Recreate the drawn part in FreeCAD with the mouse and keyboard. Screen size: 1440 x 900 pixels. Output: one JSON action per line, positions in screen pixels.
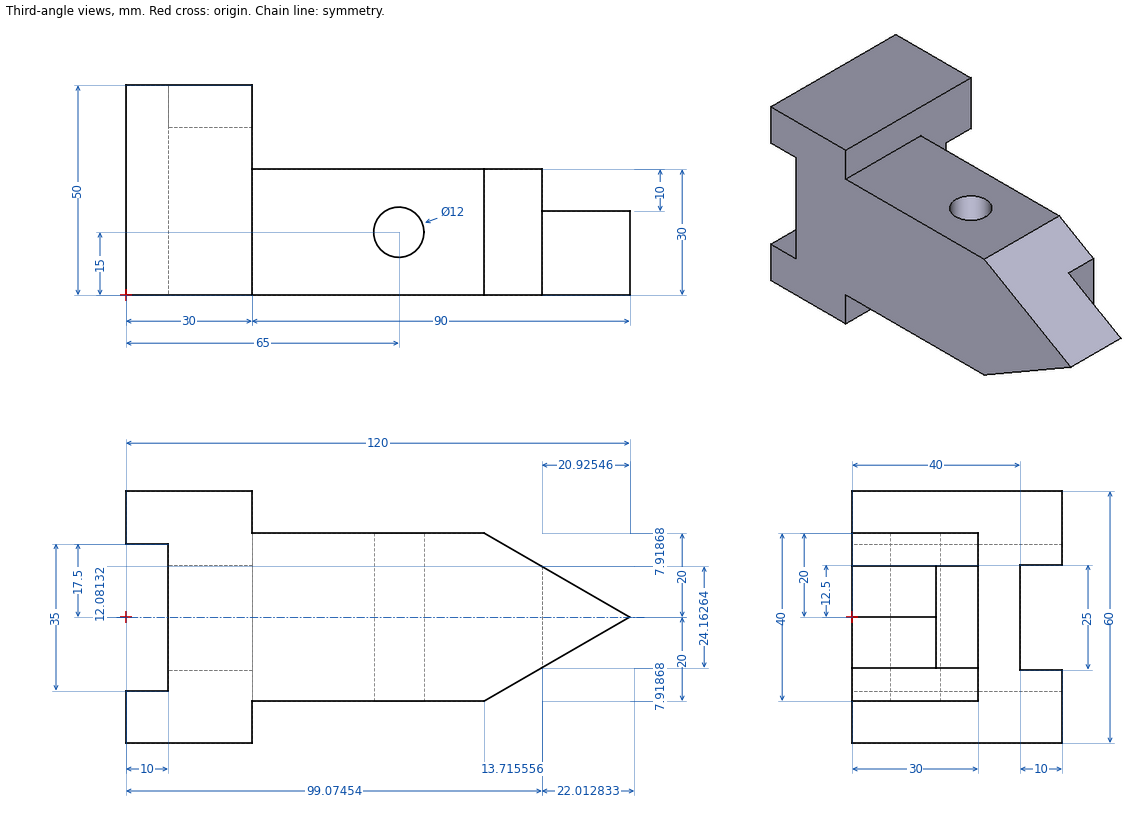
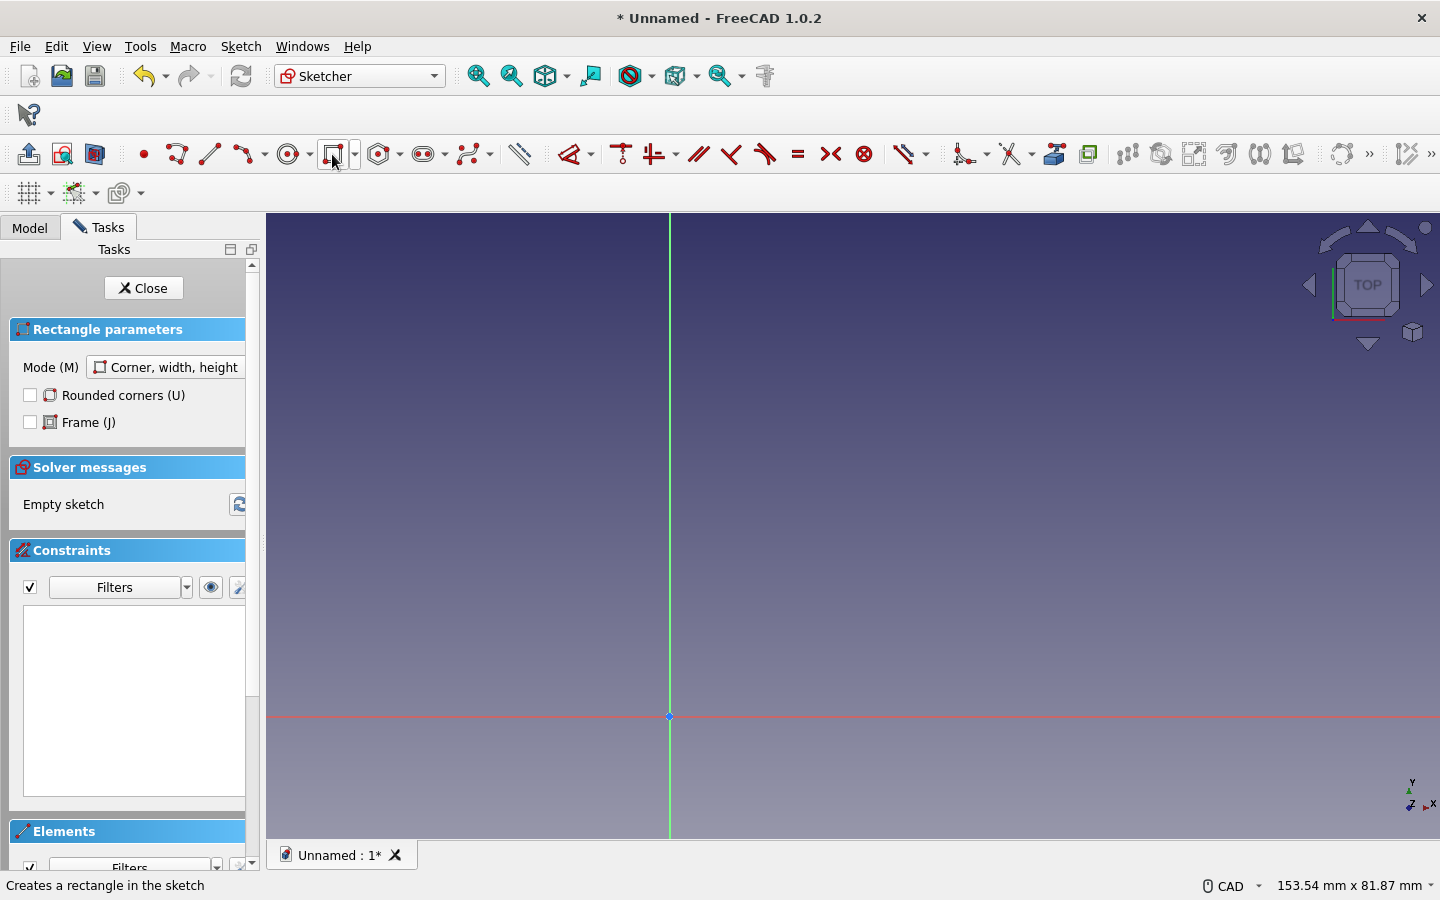
{"action": "left_click", "coordinate": [670, 717]}
{"action": "left_click", "coordinate": [899, 335]}
{"action": "key", "text": "Escape"}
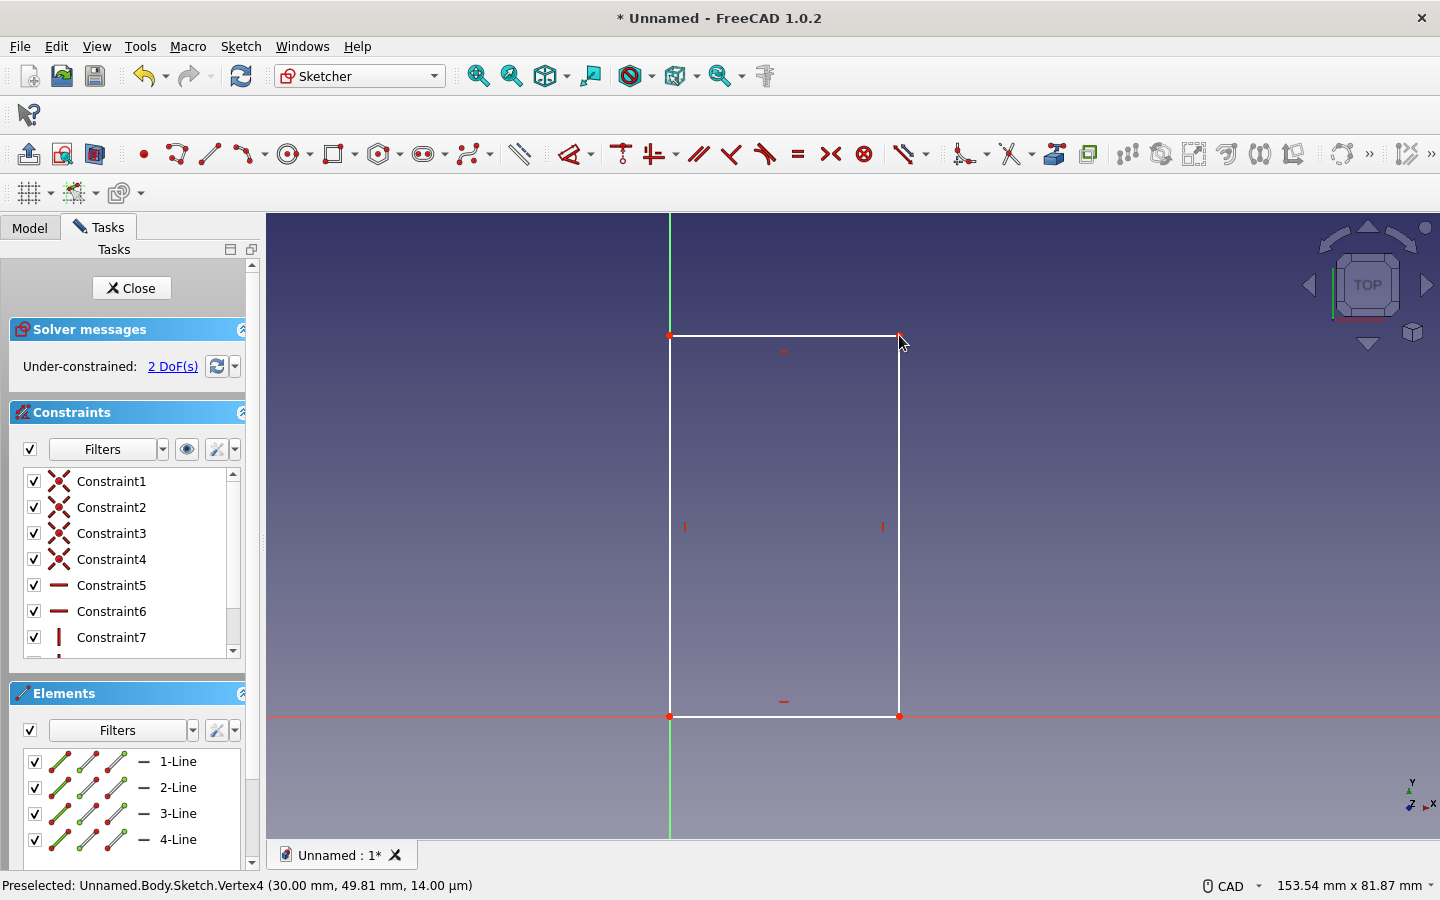
{"action": "left_click", "coordinate": [738, 717]}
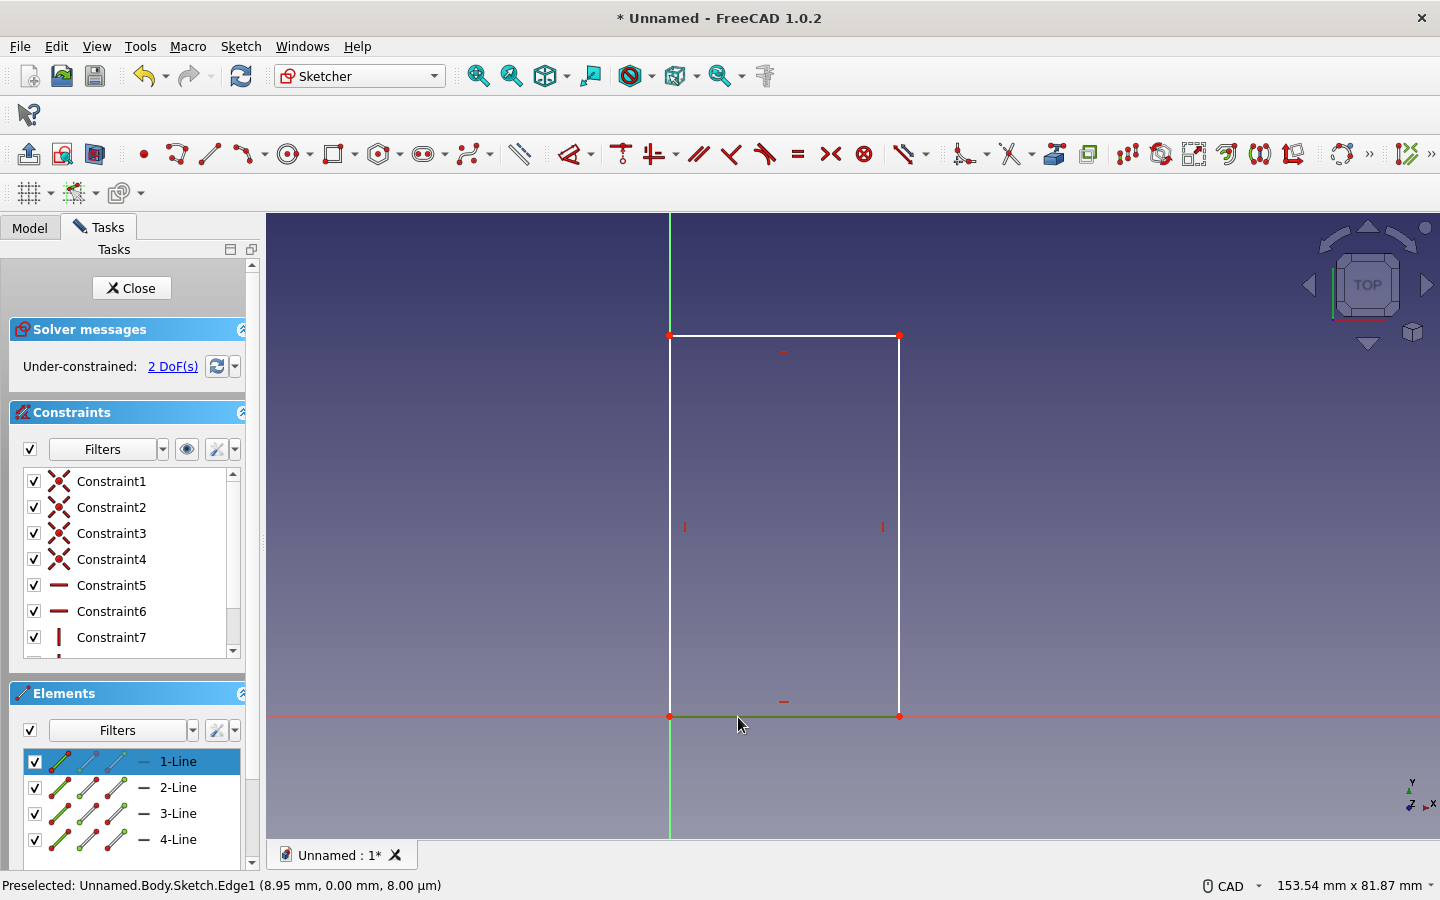
{"action": "left_click", "coordinate": [590, 154]}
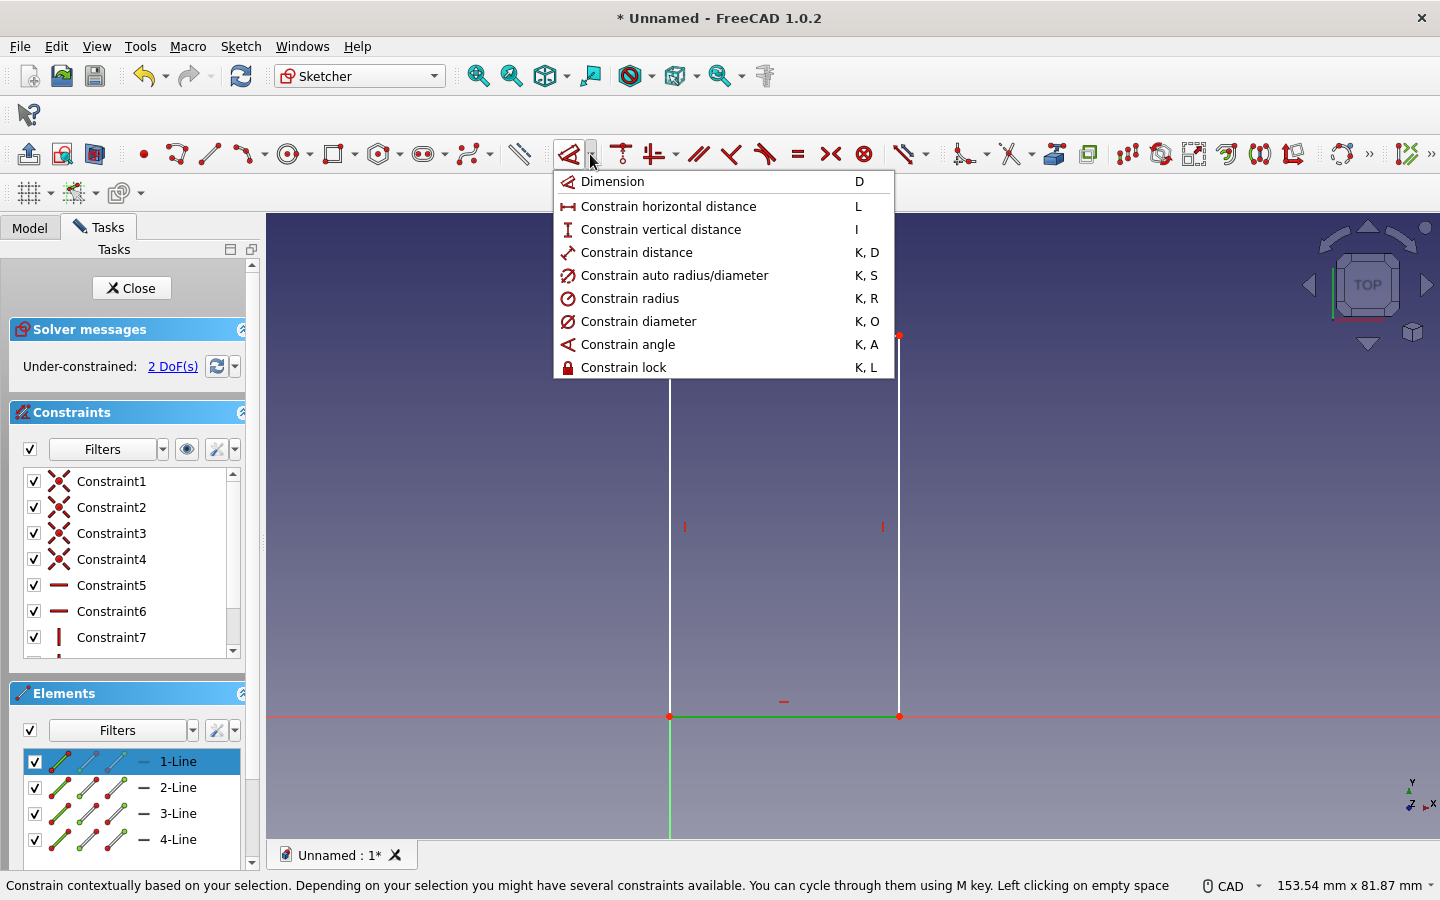
{"action": "left_click", "coordinate": [724, 206]}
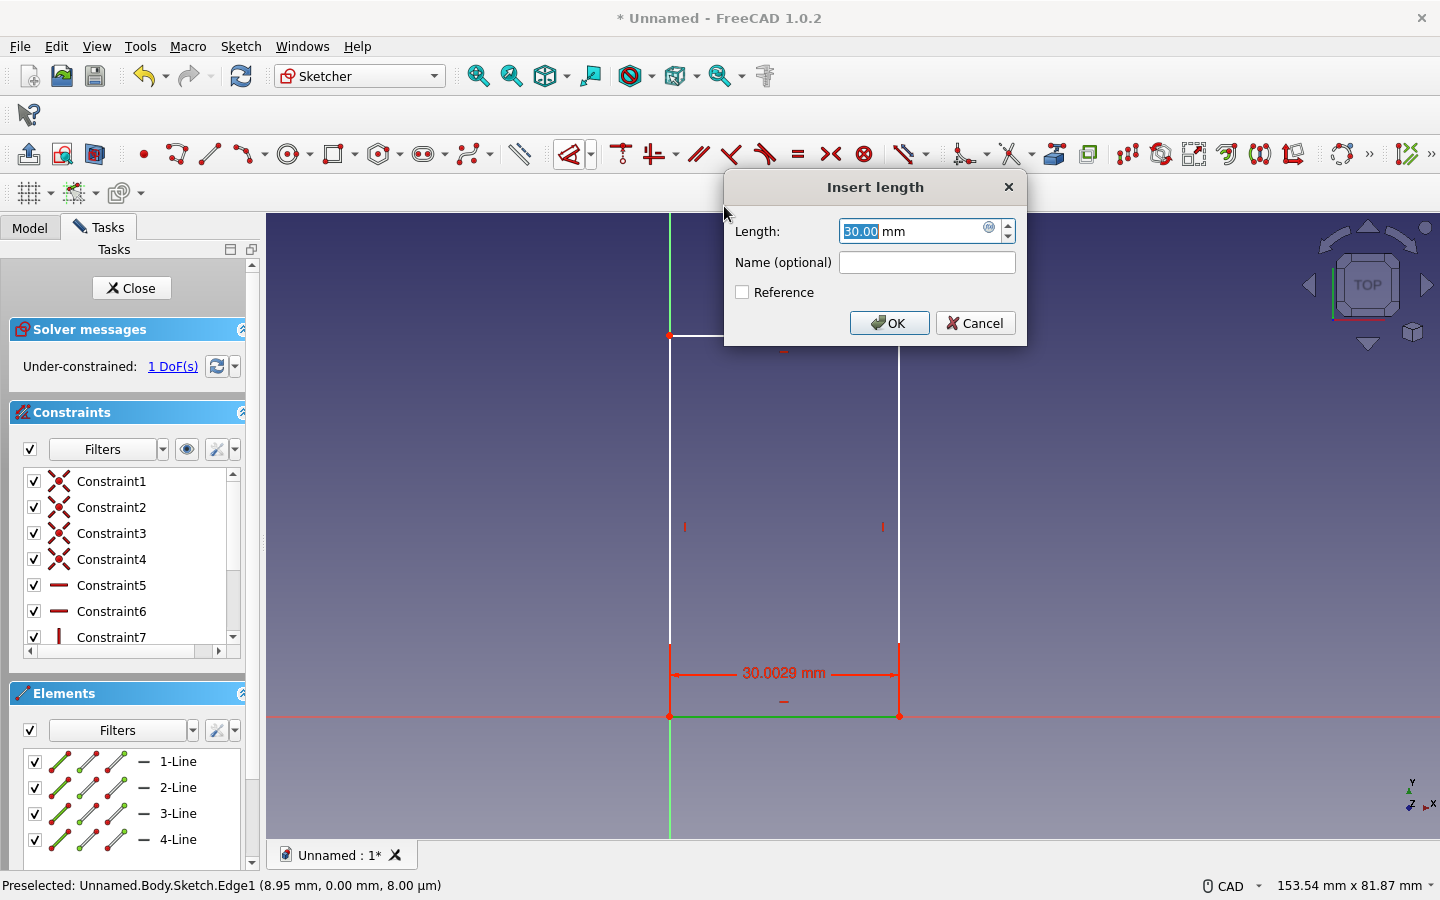
{"action": "type", "text": "30"}
{"action": "key", "text": "Return"}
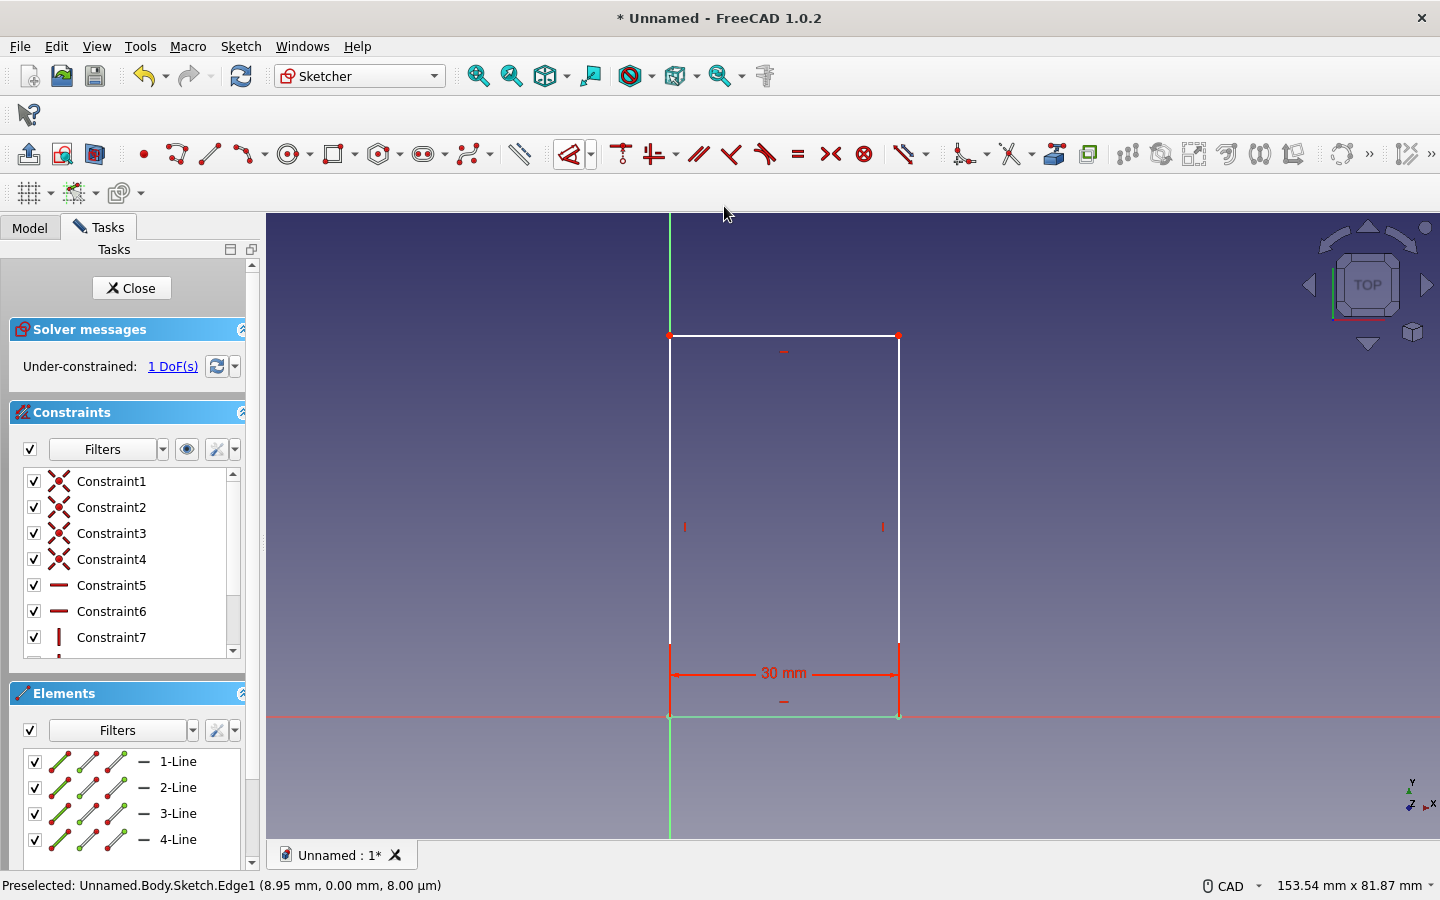
{"action": "left_click", "coordinate": [899, 603]}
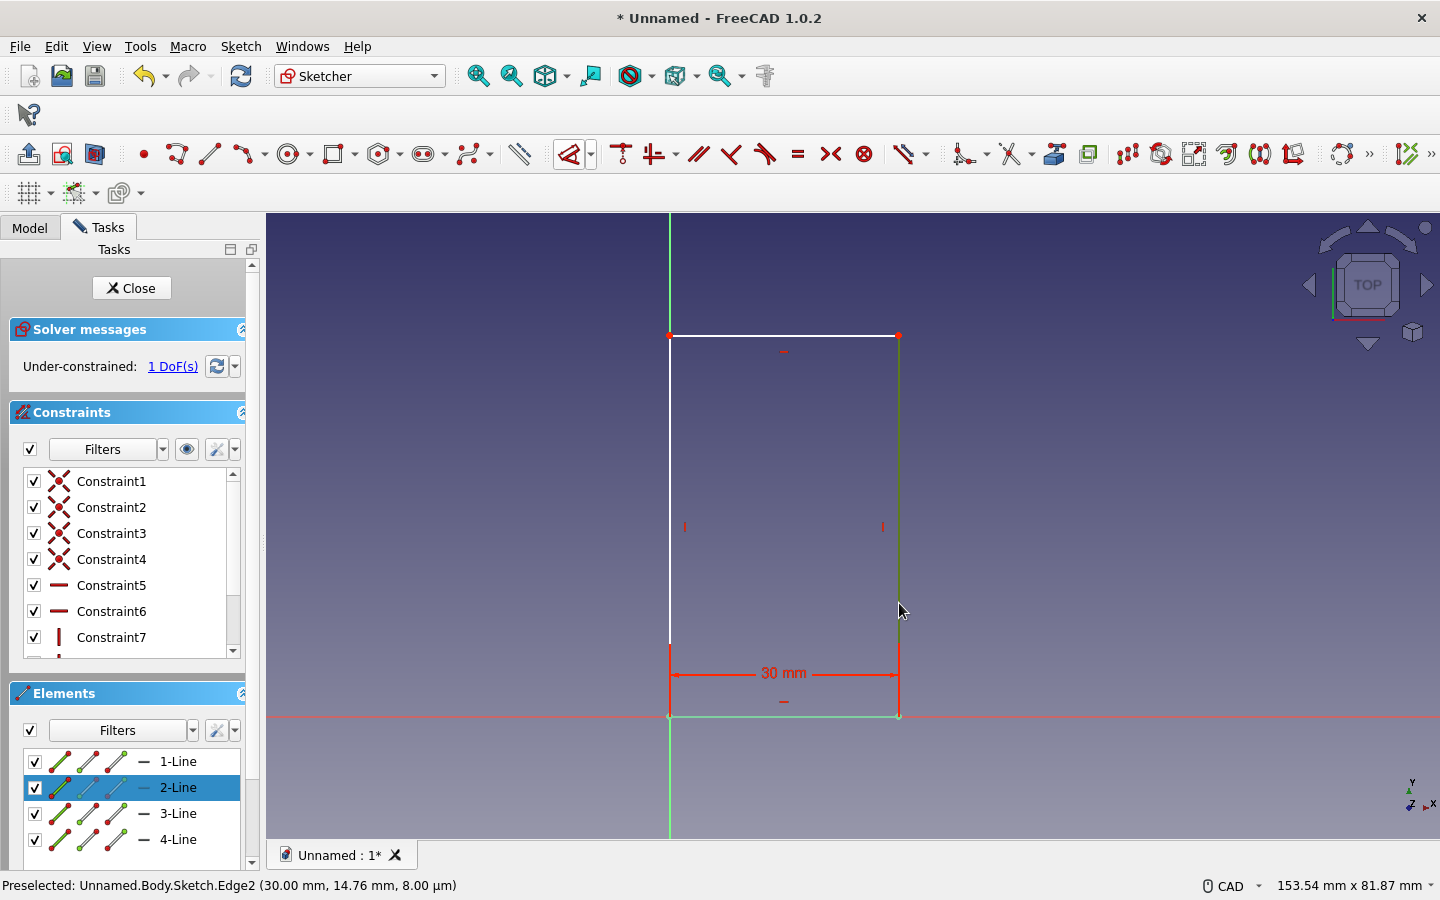
{"action": "left_click", "coordinate": [590, 154]}